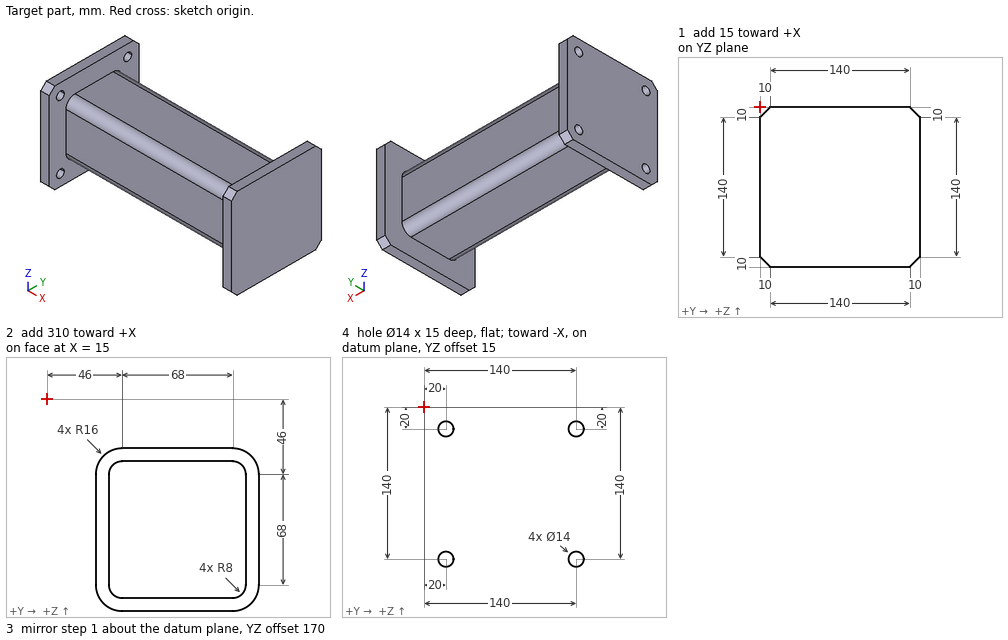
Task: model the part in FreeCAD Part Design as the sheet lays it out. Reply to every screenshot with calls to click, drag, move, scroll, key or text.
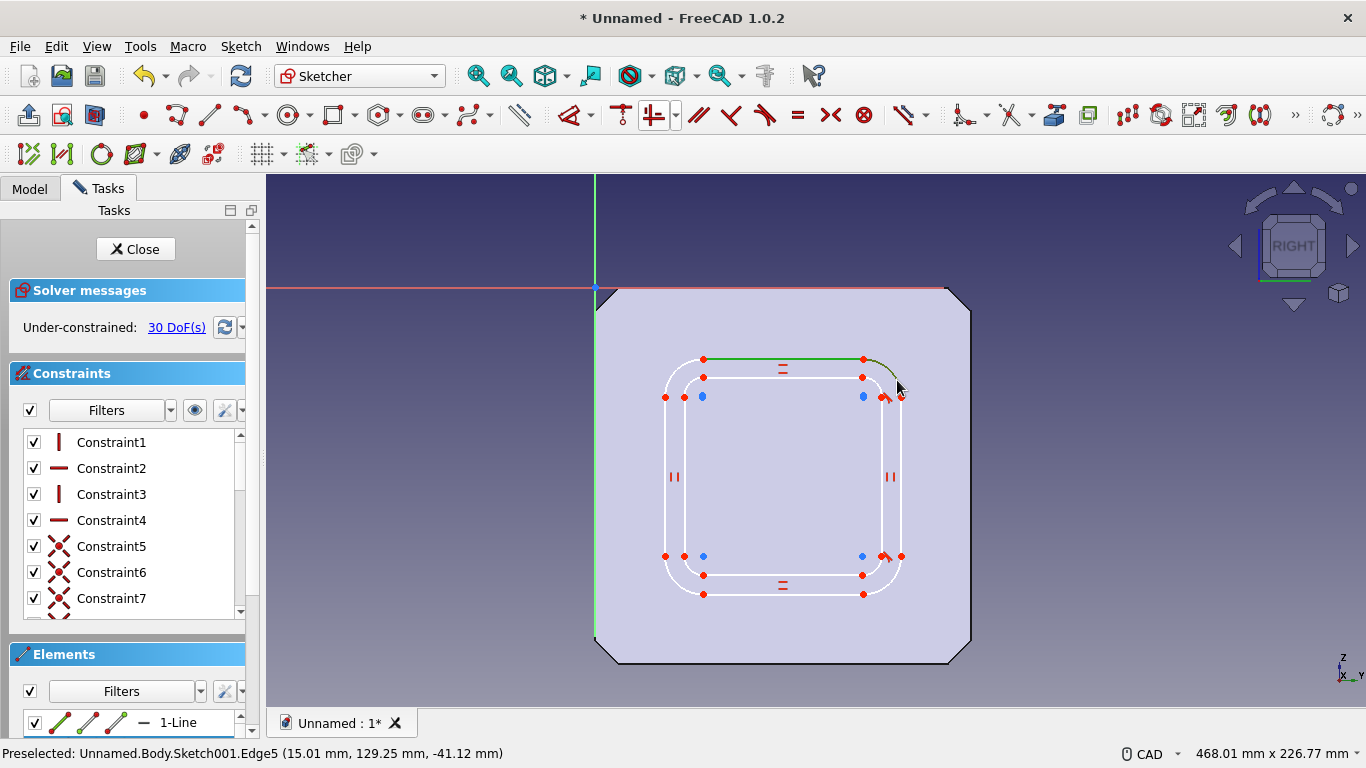
click(765, 116)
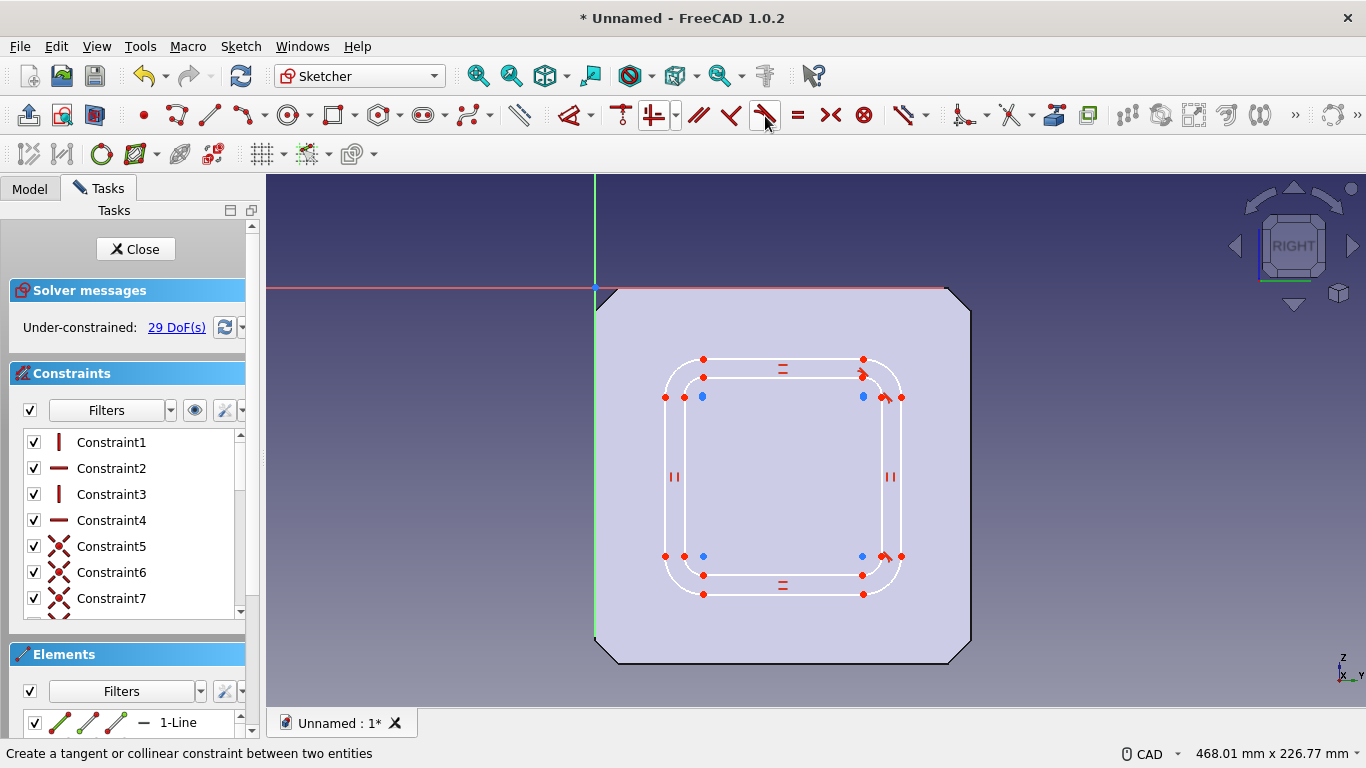
click(815, 359)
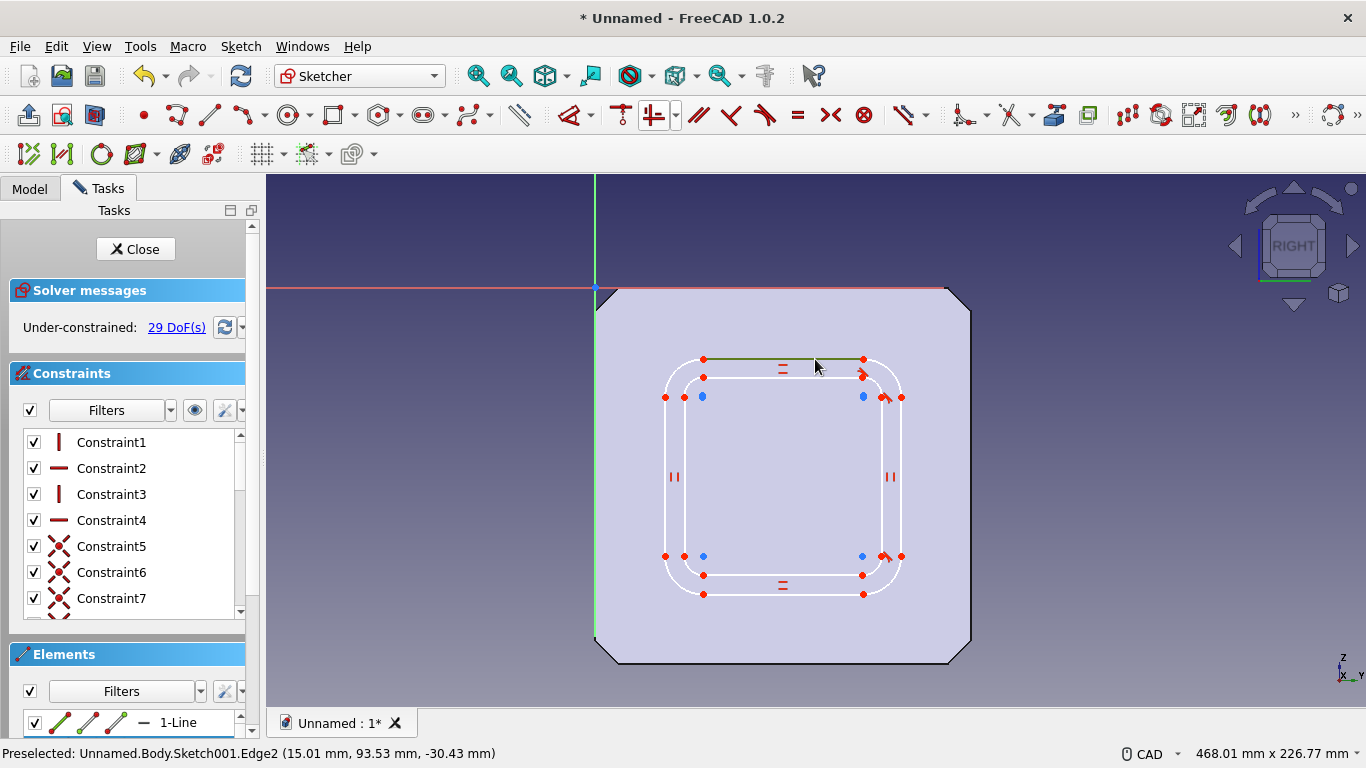
click(686, 363)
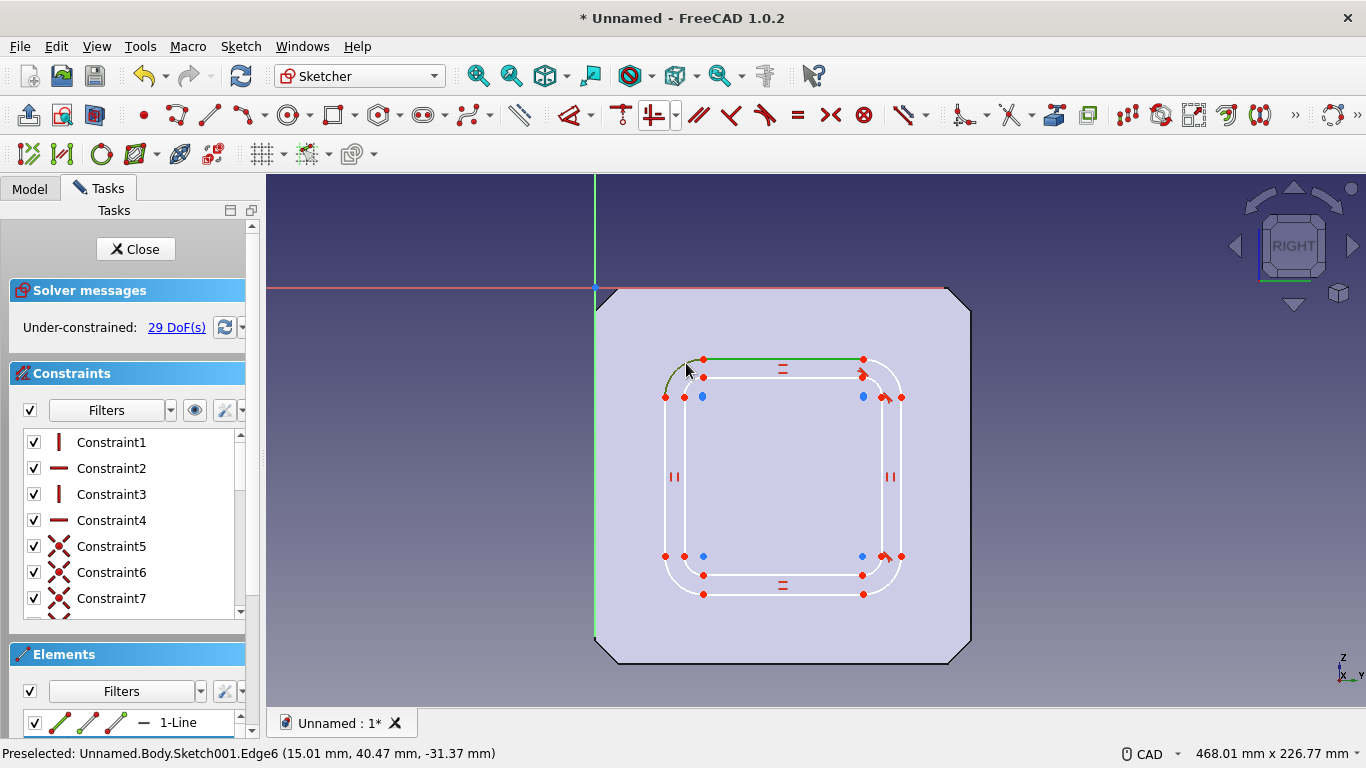
click(765, 116)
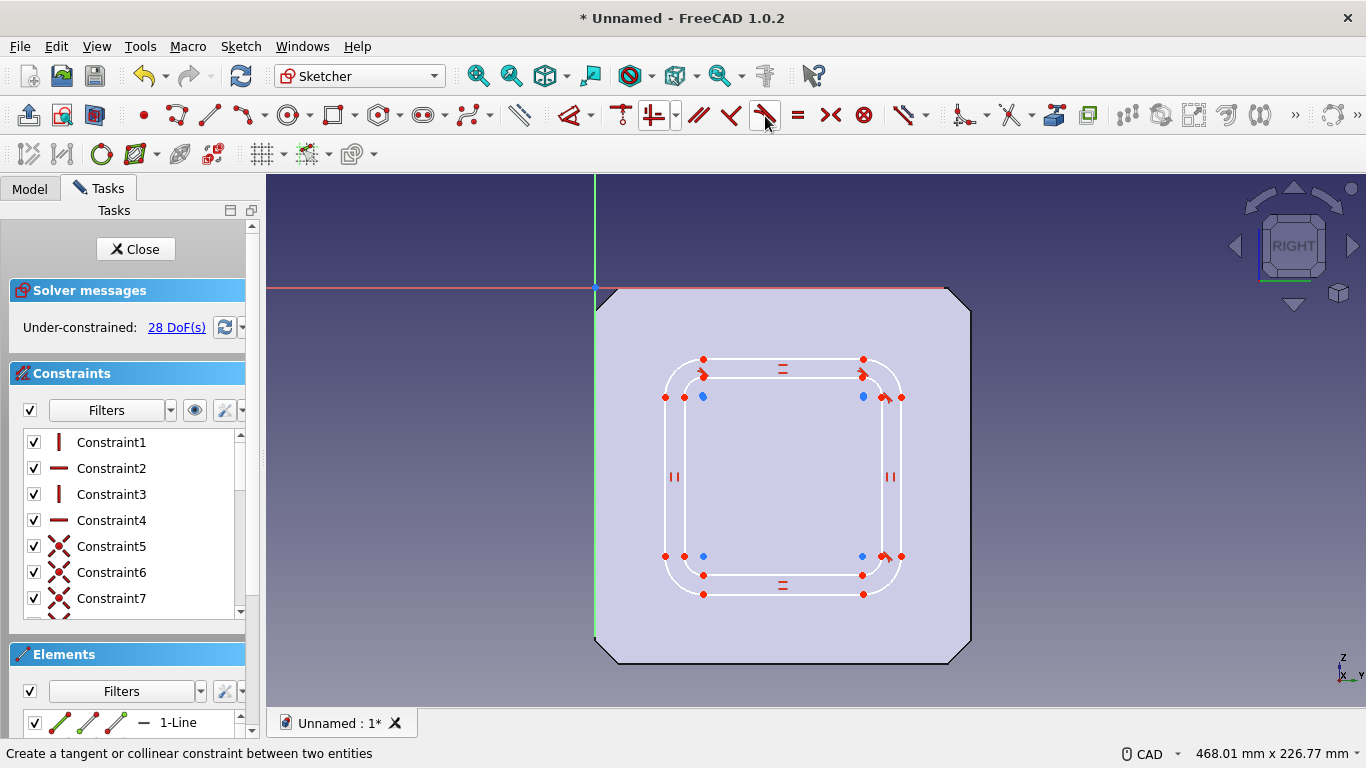
click(665, 445)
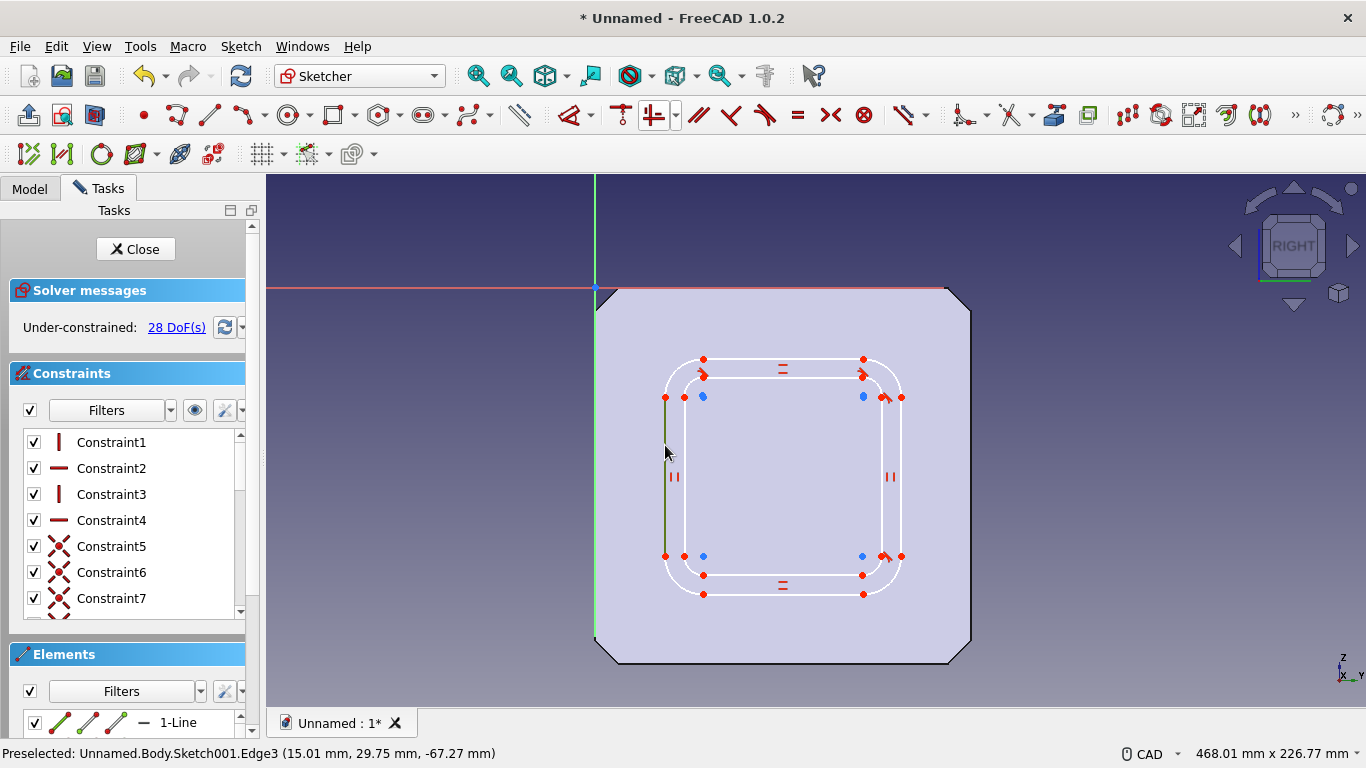
click(686, 363)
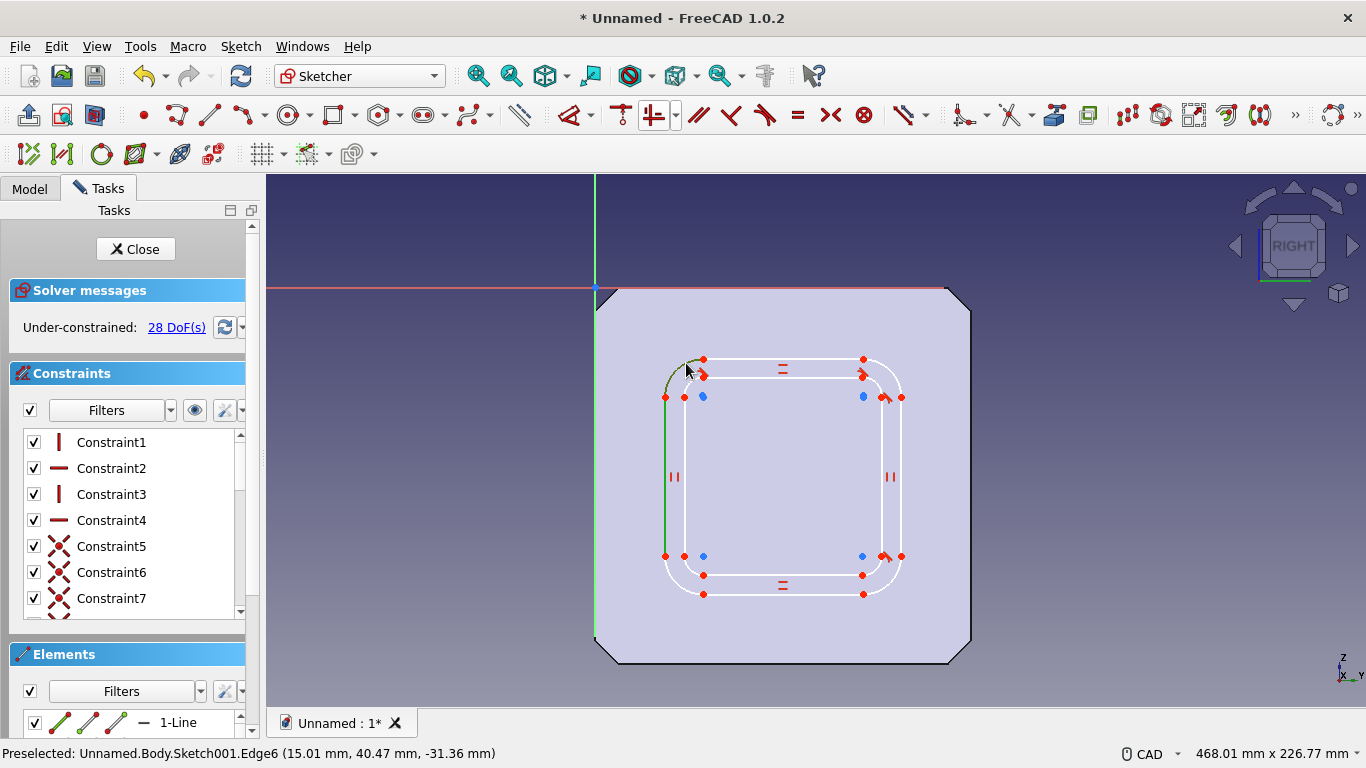
click(765, 116)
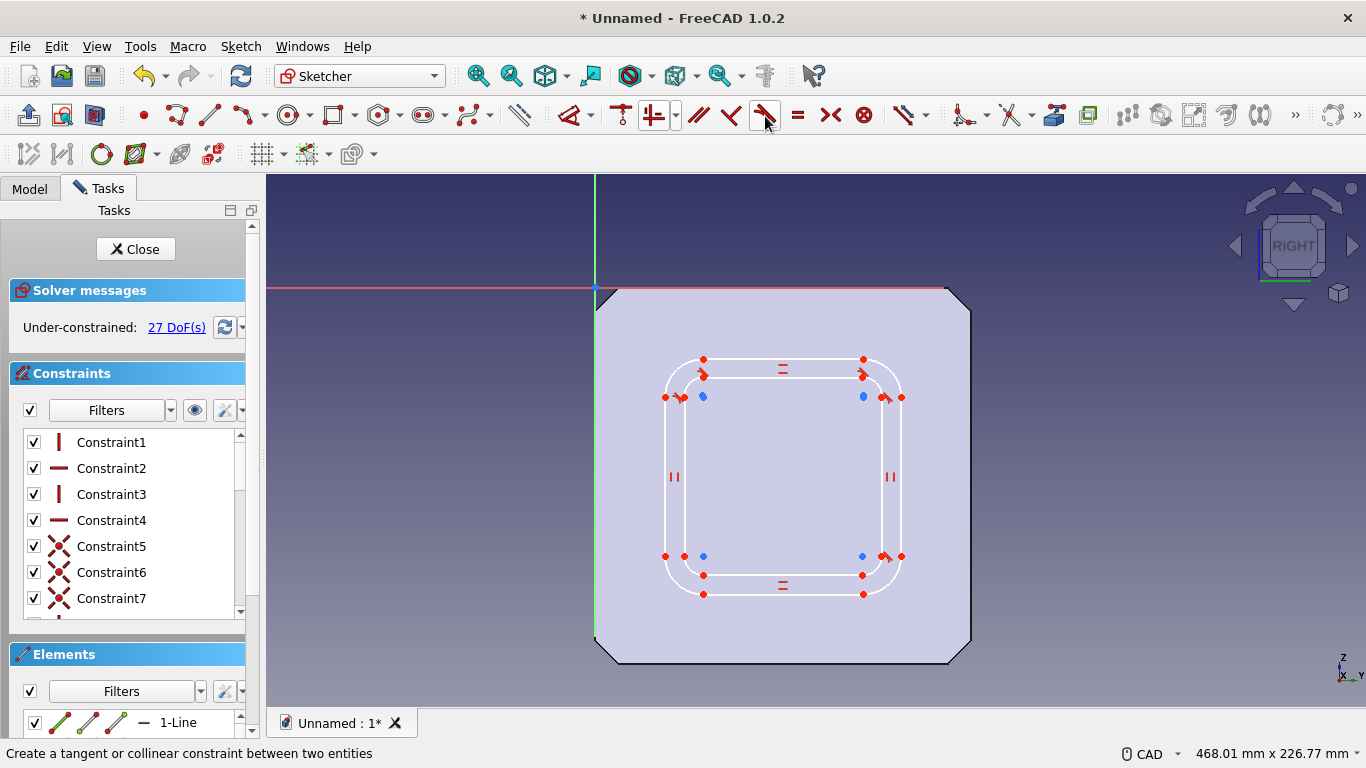
click(665, 445)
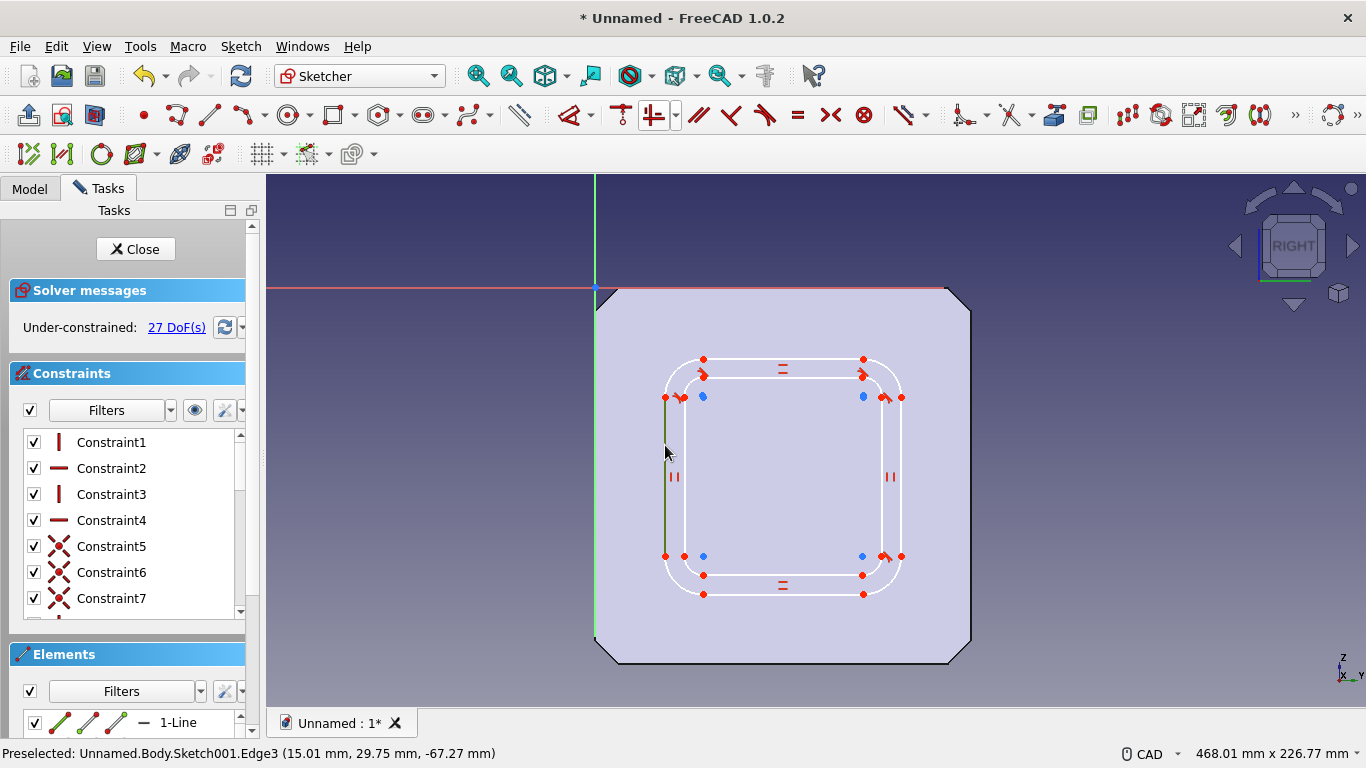
click(669, 574)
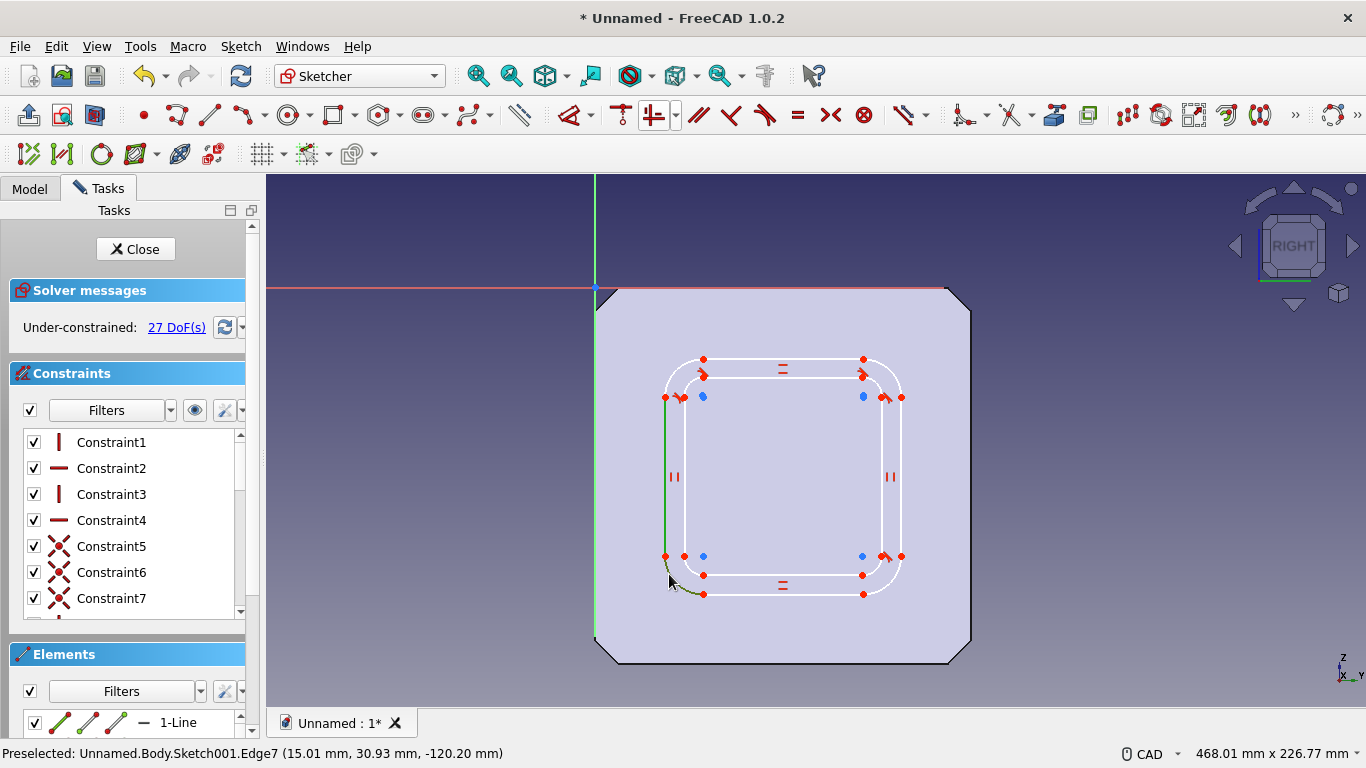
click(765, 116)